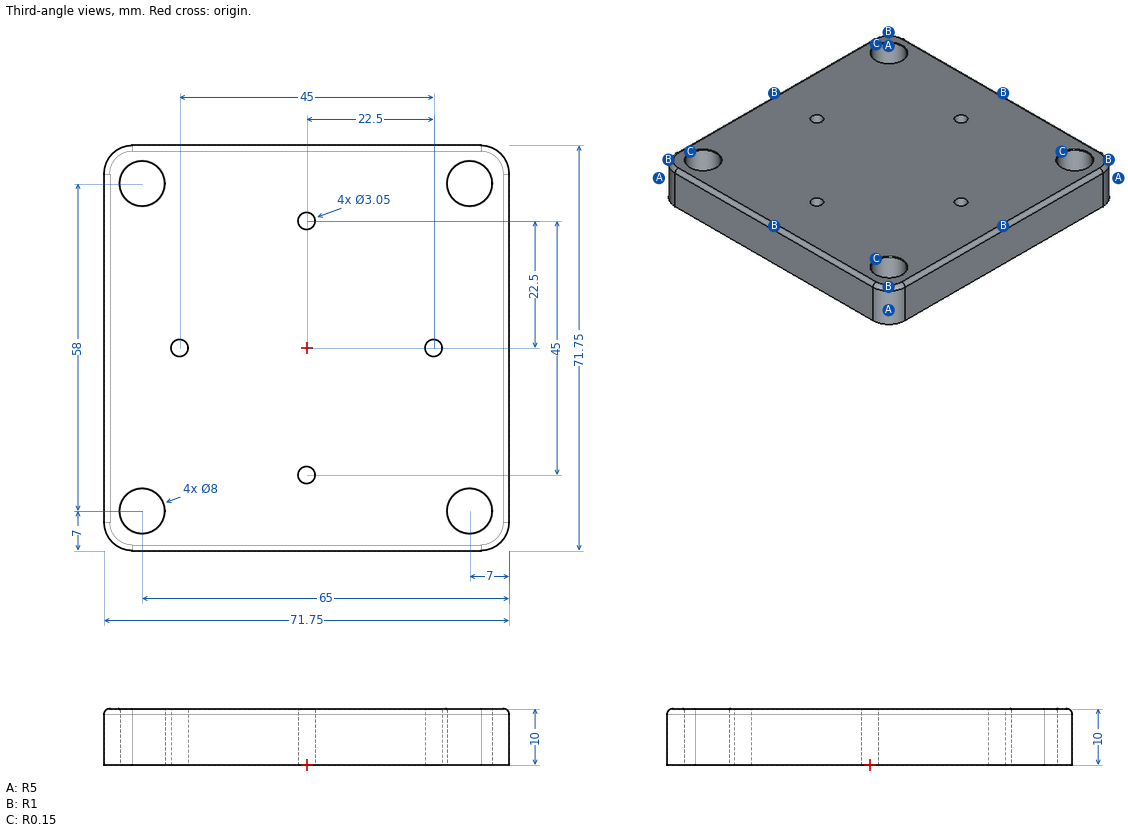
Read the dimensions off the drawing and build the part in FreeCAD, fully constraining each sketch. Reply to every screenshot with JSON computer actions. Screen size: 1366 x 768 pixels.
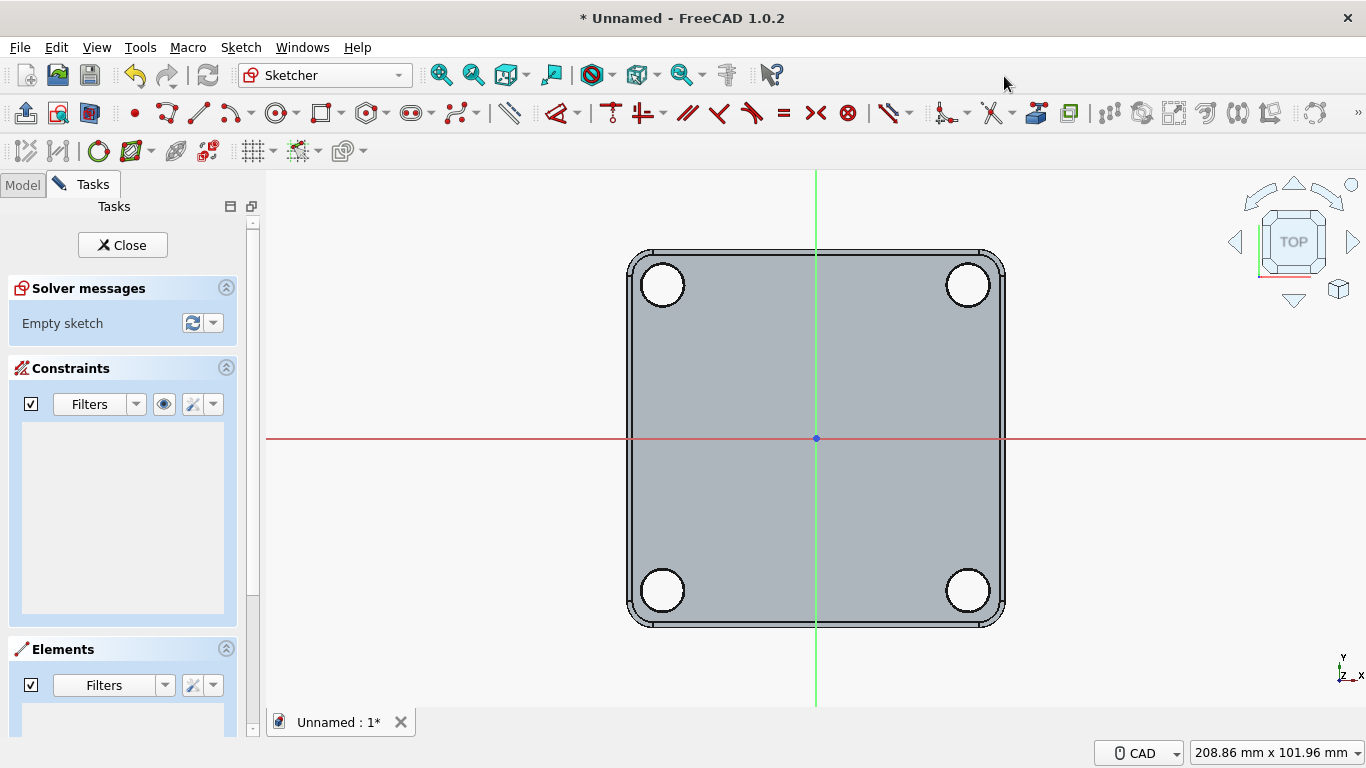
{"action": "left_click", "coordinate": [276, 114]}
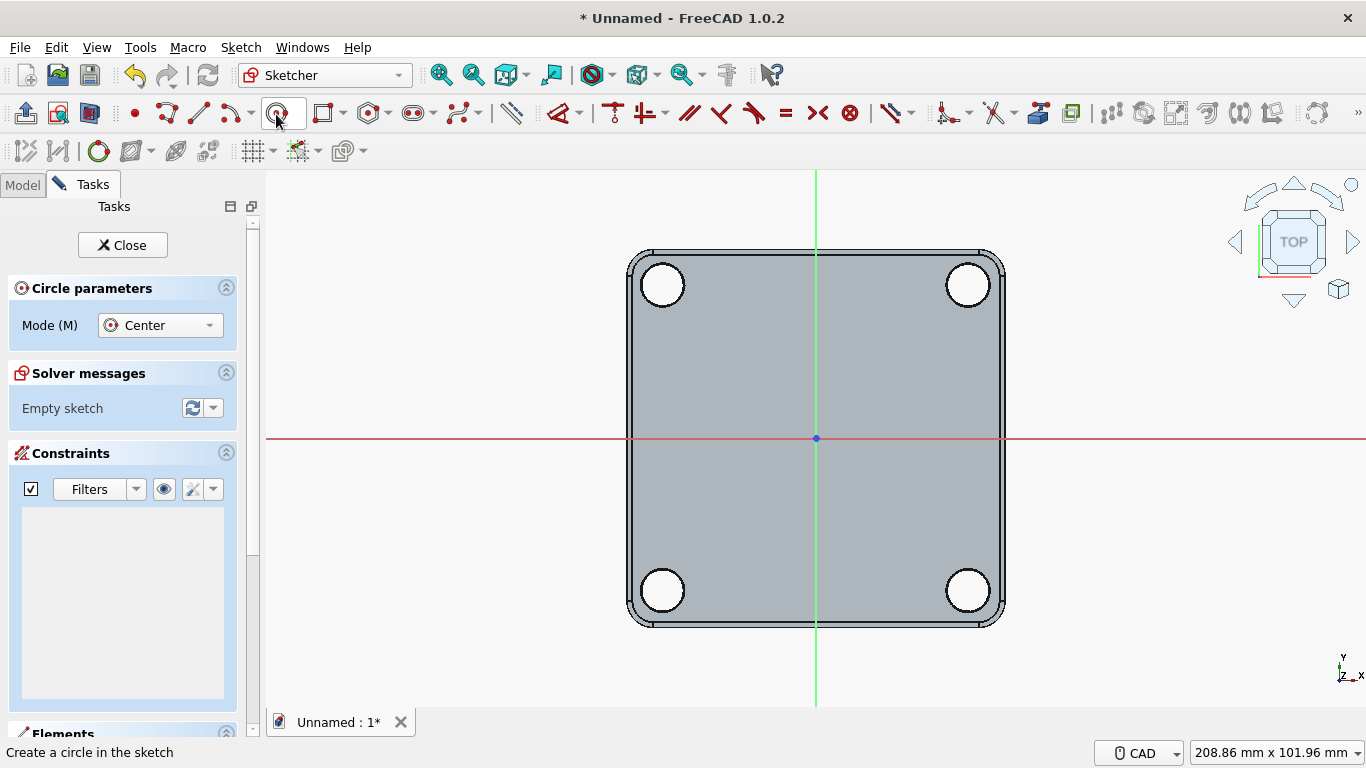
{"action": "scroll", "coordinate": [816, 320], "scroll_direction": "up", "scroll_amount": 6}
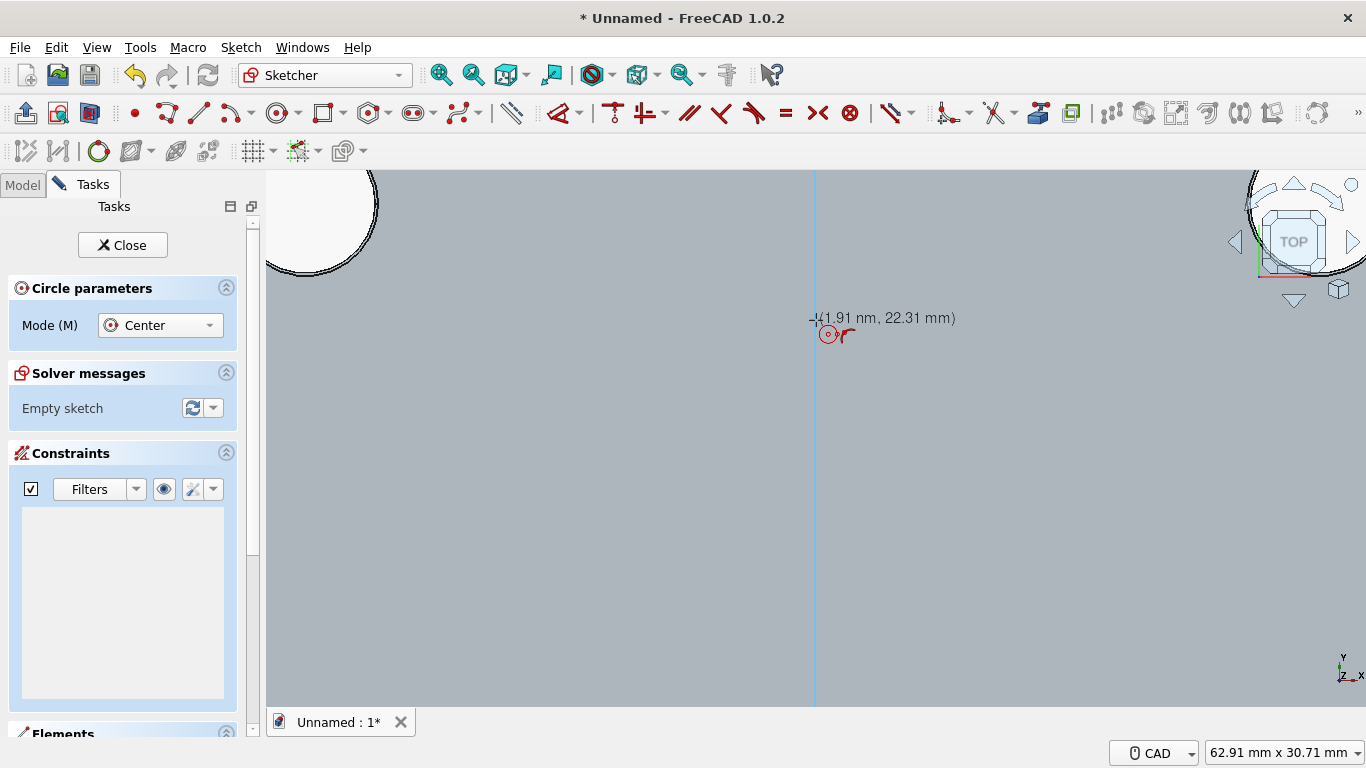
{"action": "left_click", "coordinate": [815, 319]}
{"action": "left_click", "coordinate": [834, 300]}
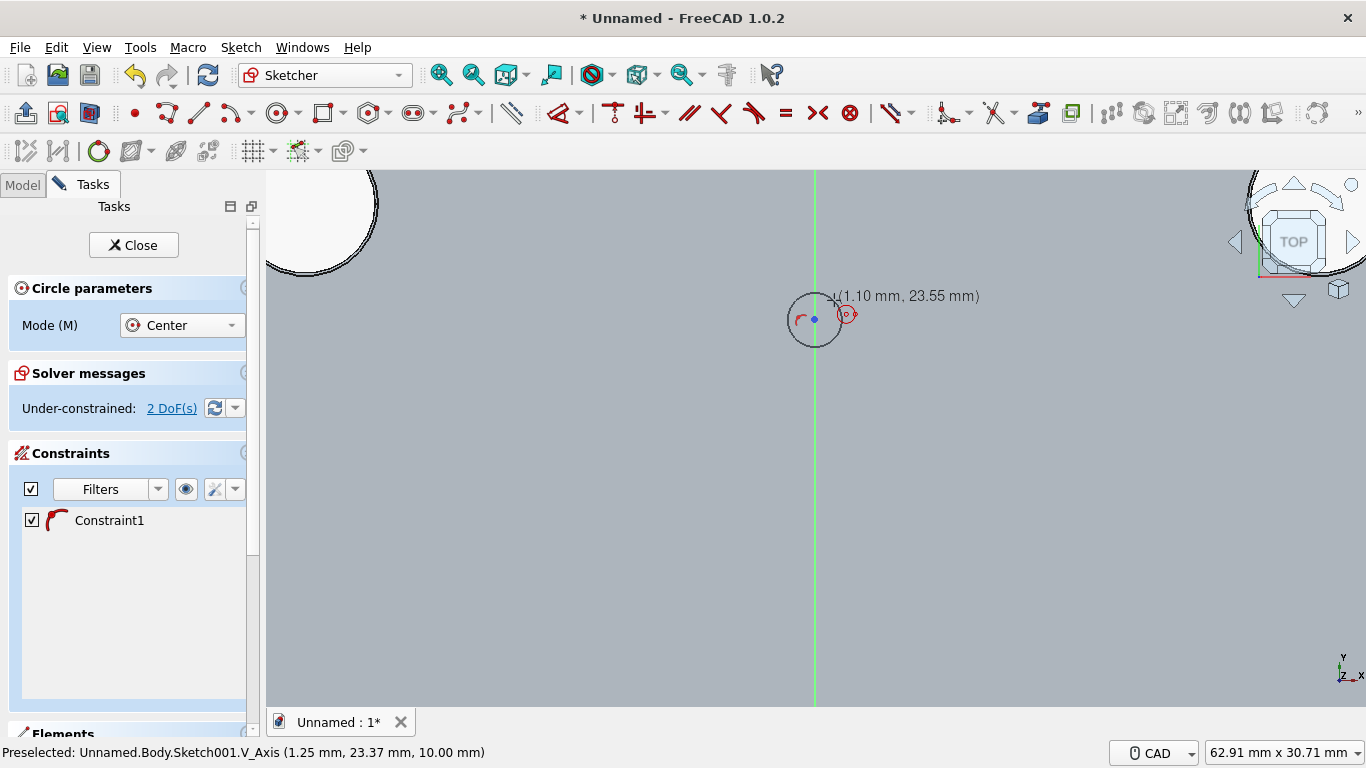
{"action": "scroll", "coordinate": [708, 279], "scroll_direction": "down", "scroll_amount": 5}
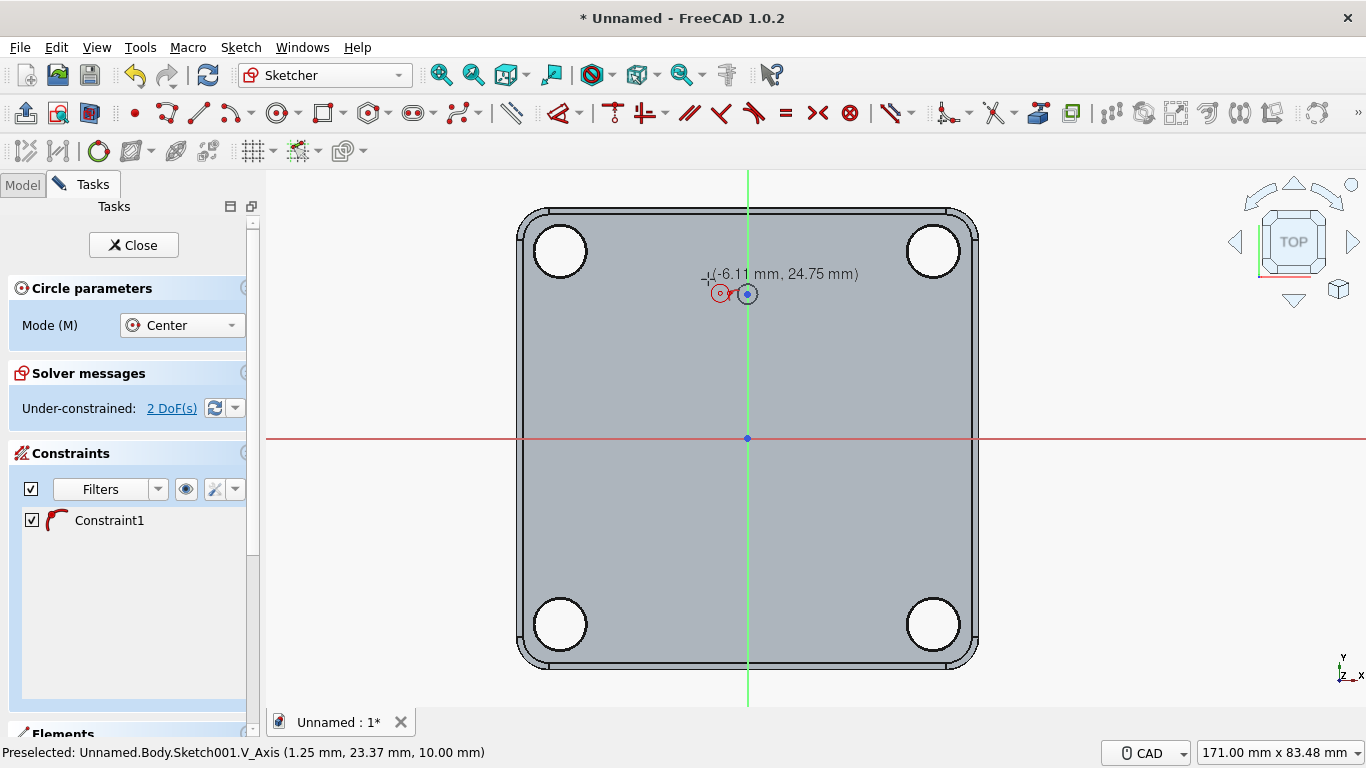
{"action": "scroll", "coordinate": [892, 439], "scroll_direction": "up", "scroll_amount": 5}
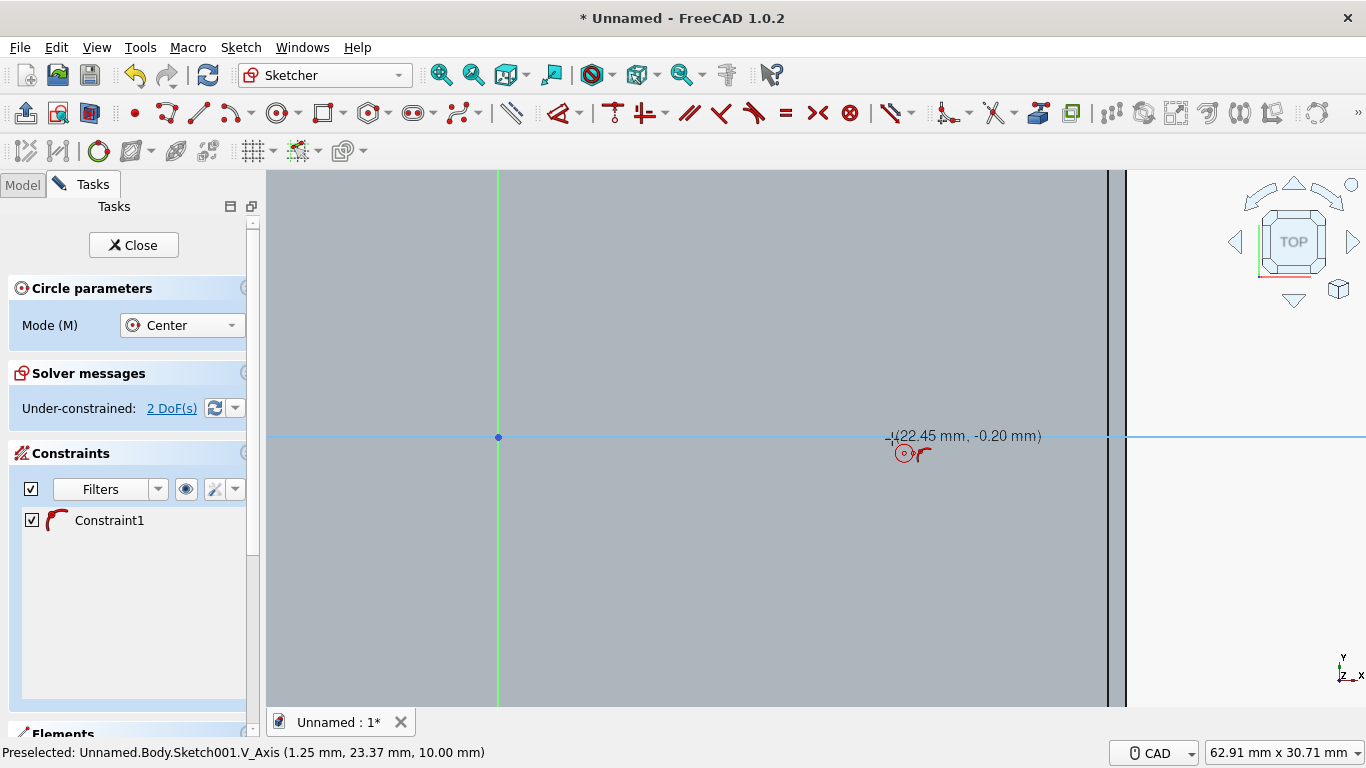
{"action": "left_click", "coordinate": [892, 437]}
{"action": "left_click", "coordinate": [911, 418]}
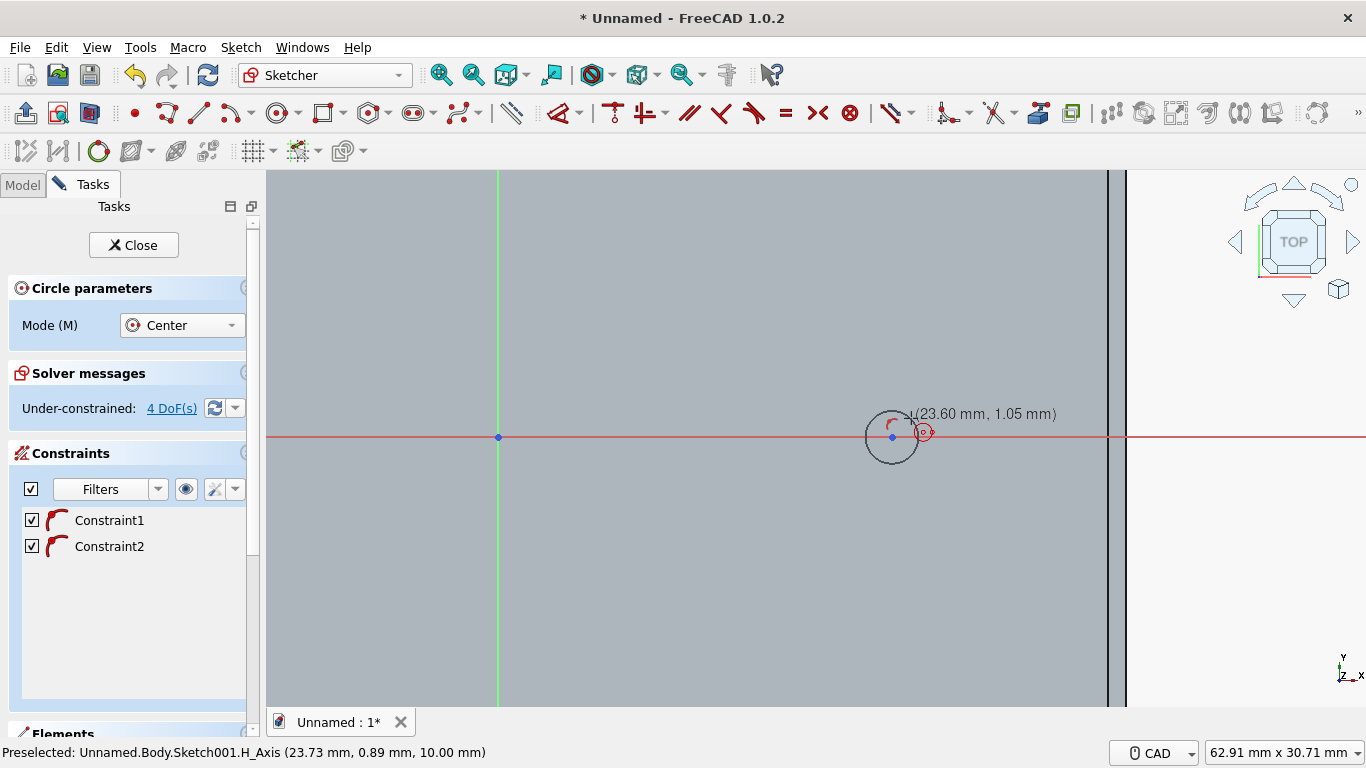
{"action": "scroll", "coordinate": [892, 439], "scroll_direction": "down", "scroll_amount": 5}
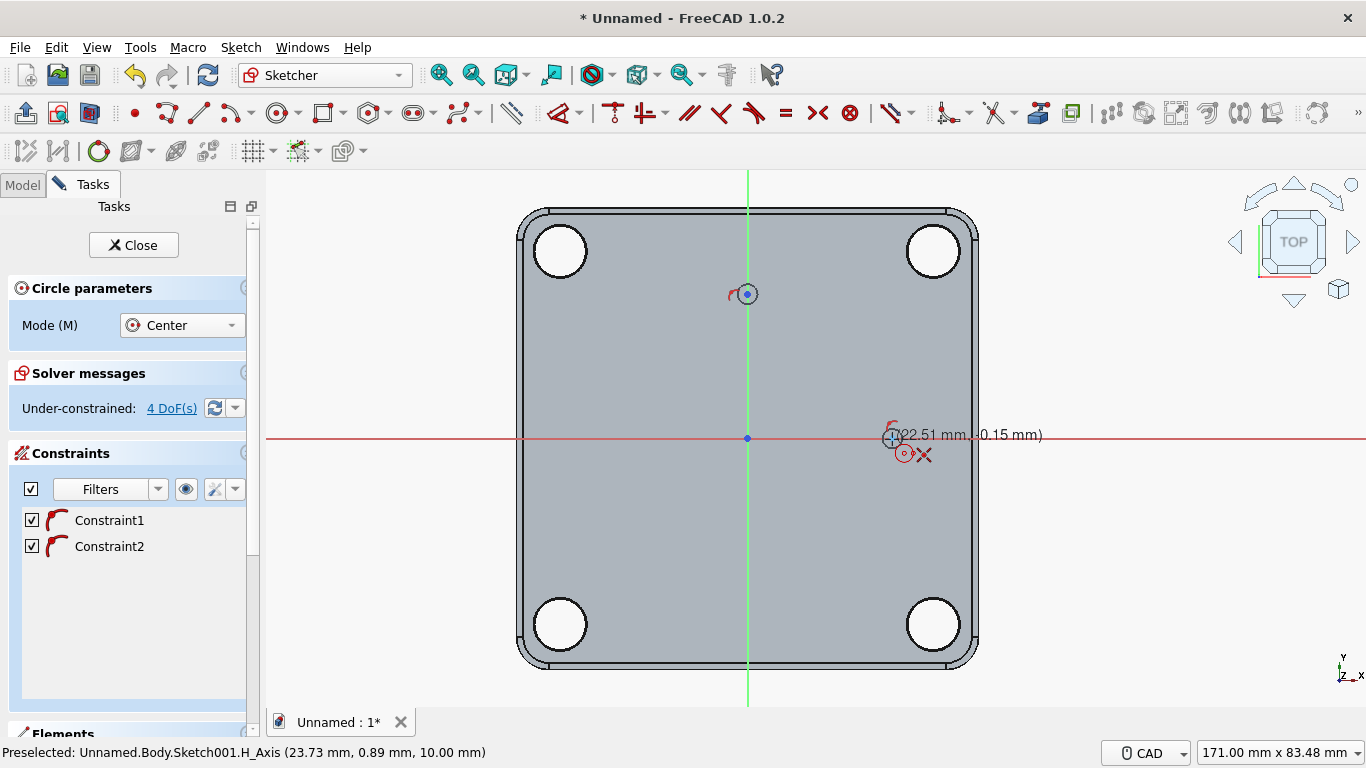
{"action": "scroll", "coordinate": [748, 583], "scroll_direction": "up", "scroll_amount": 5}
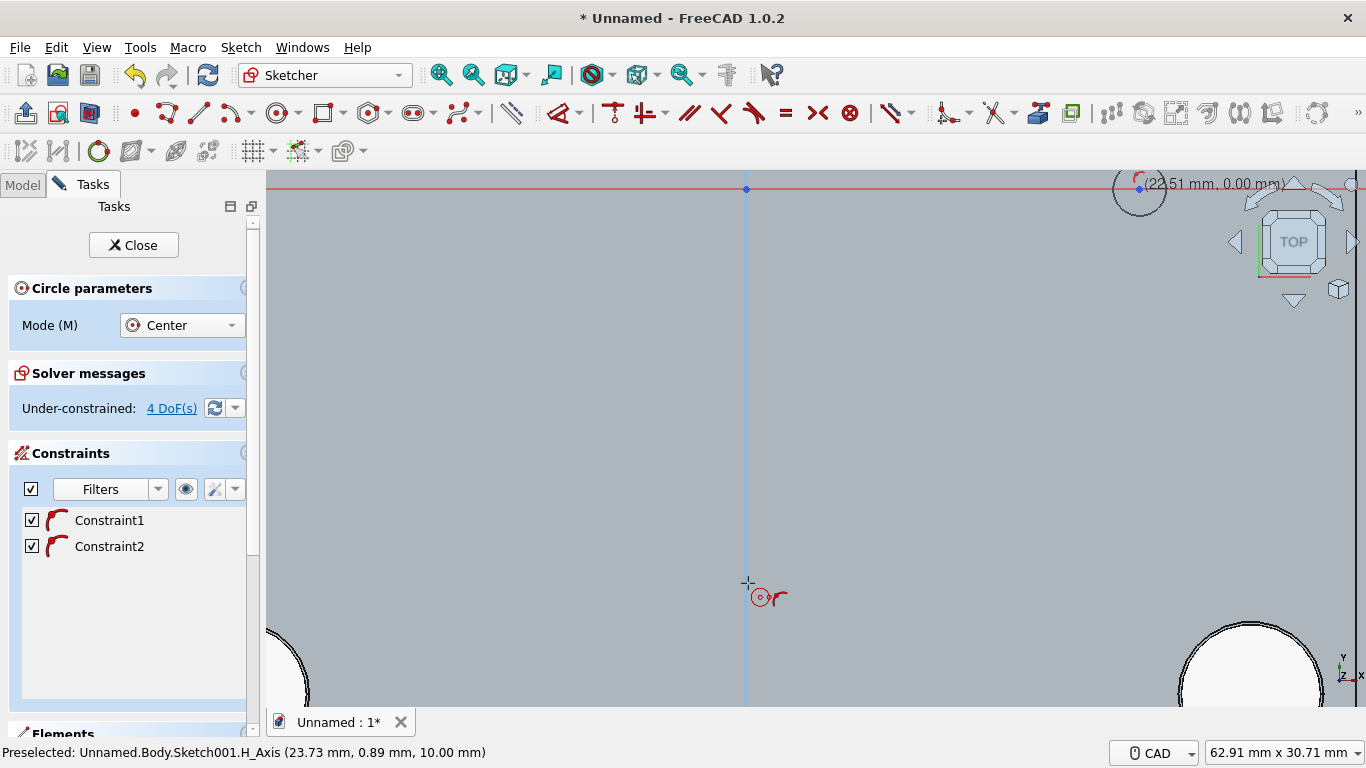
{"action": "left_click", "coordinate": [746, 583]}
{"action": "left_click", "coordinate": [765, 564]}